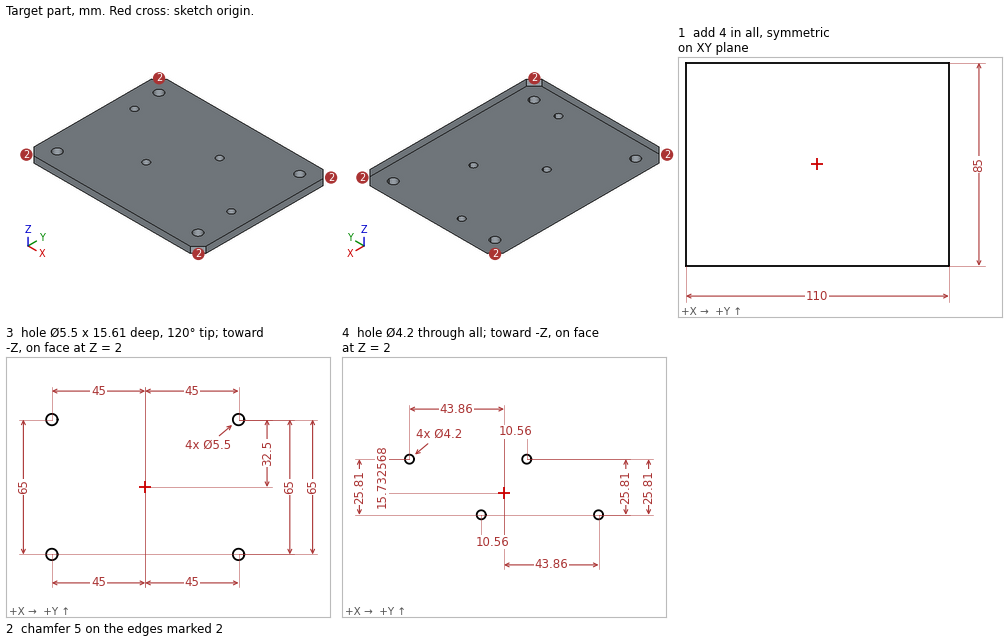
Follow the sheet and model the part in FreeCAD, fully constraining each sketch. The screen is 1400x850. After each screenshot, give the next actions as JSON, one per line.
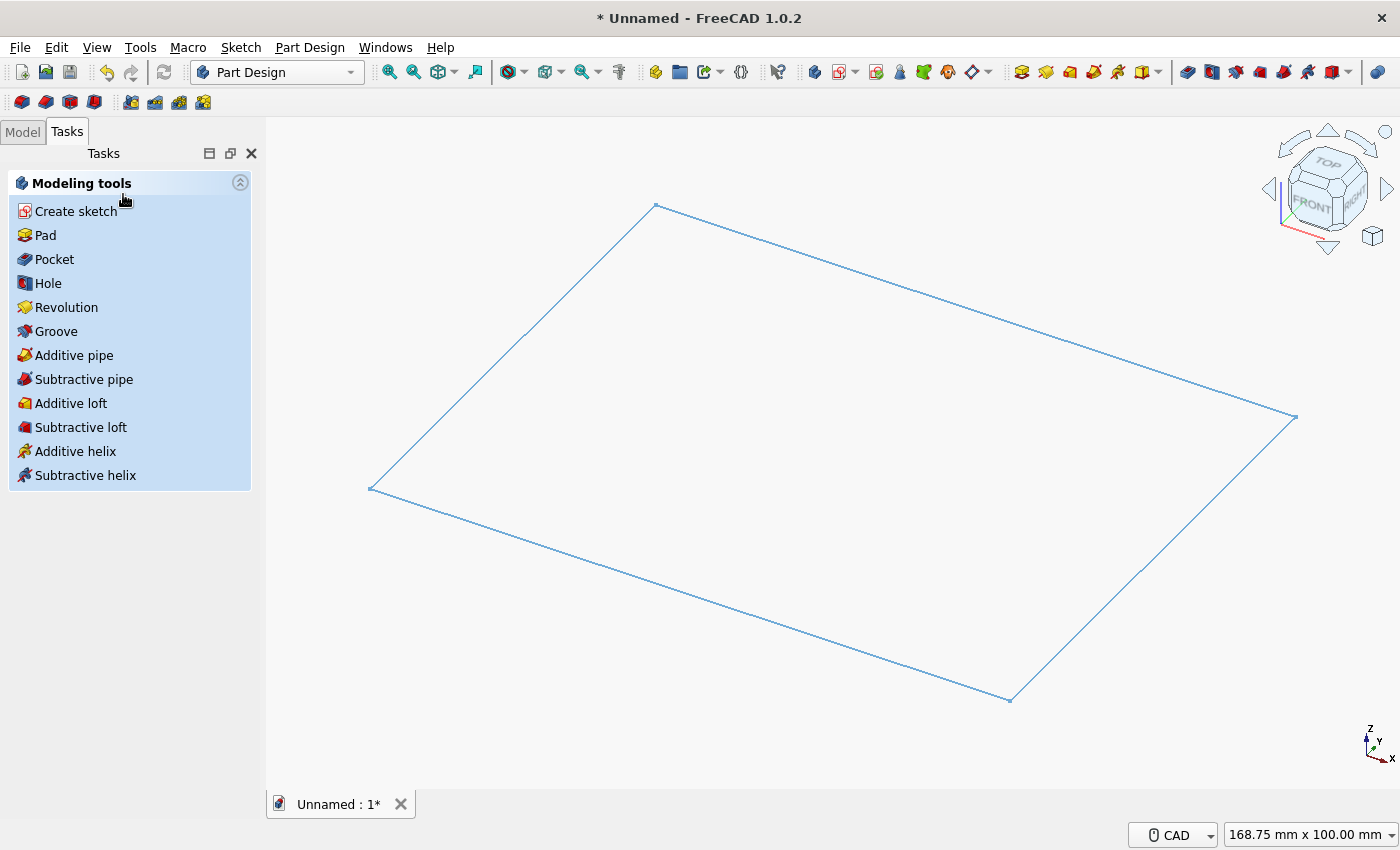
{"action": "left_click", "coordinate": [1022, 72]}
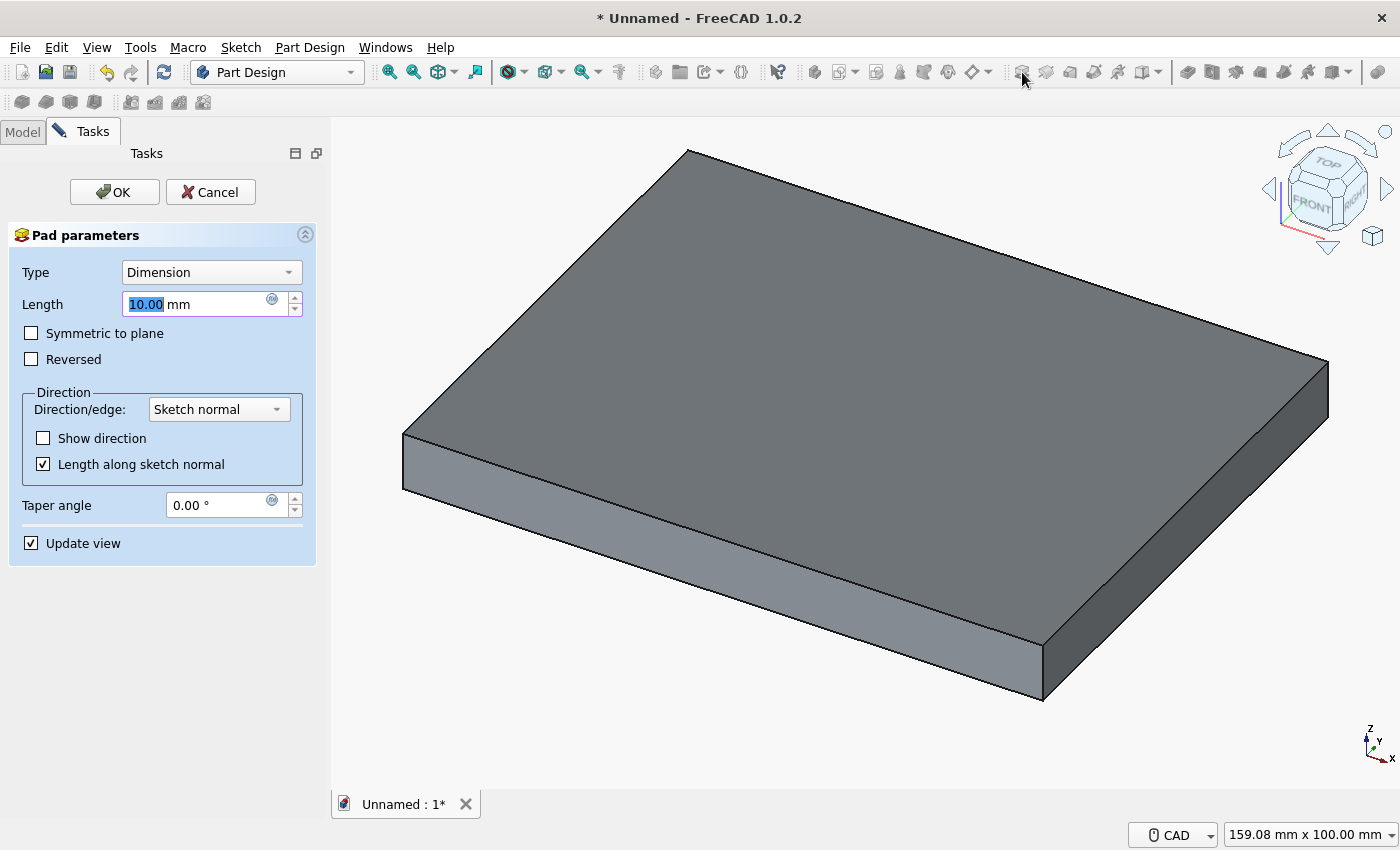
{"action": "type", "text": "4"}
{"action": "key", "text": "Tab"}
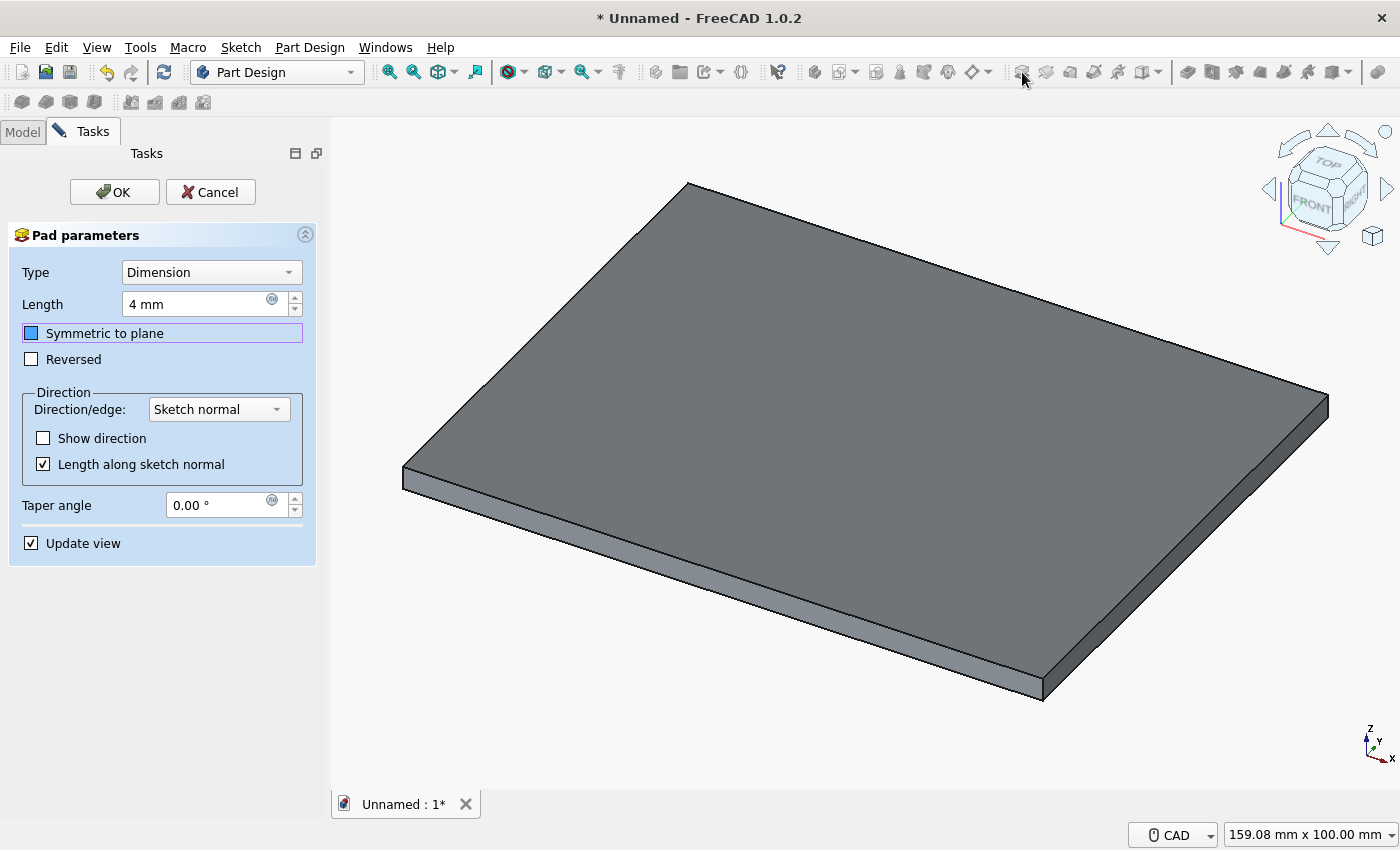
{"action": "left_click", "coordinate": [30, 333]}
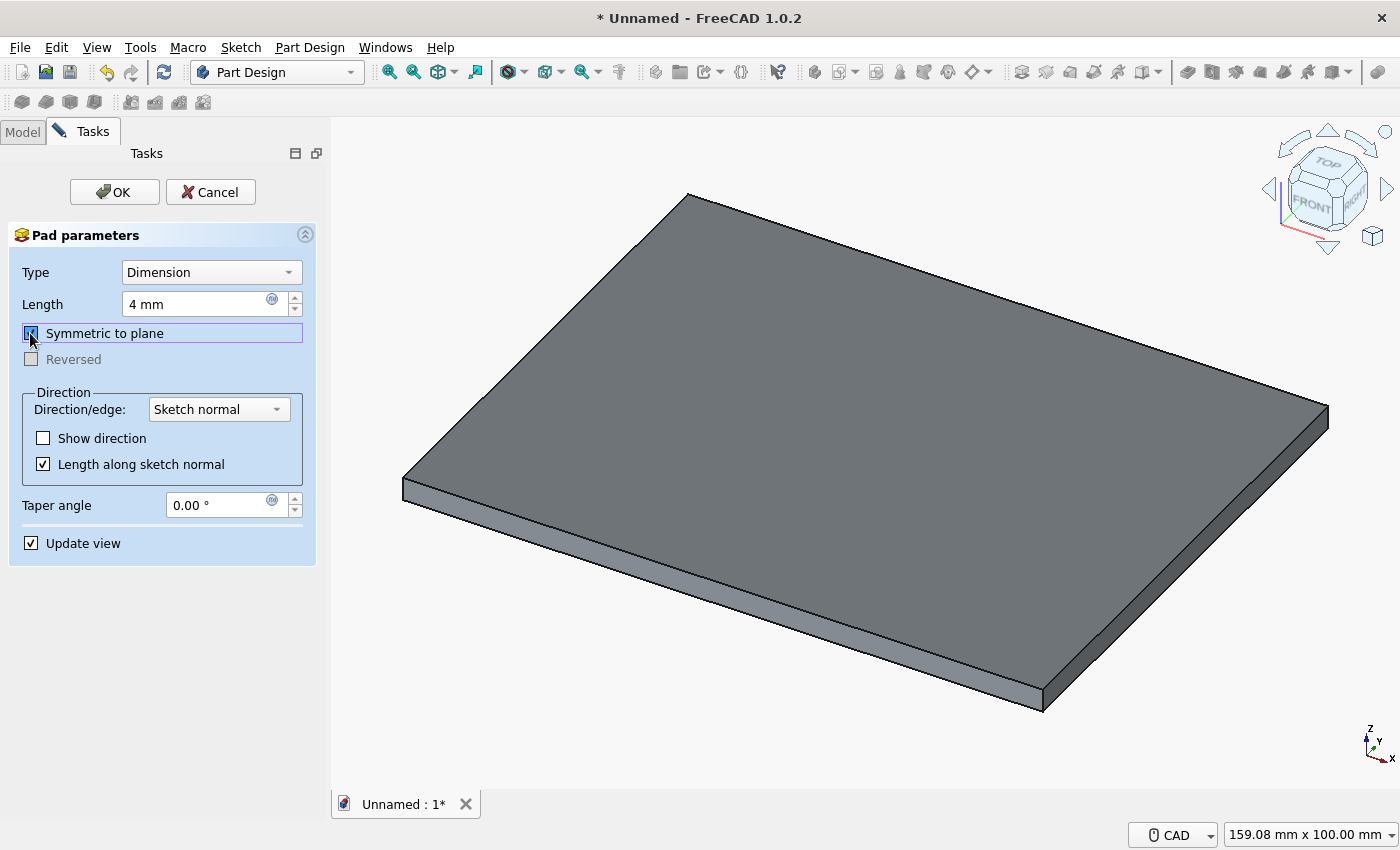
{"action": "left_click", "coordinate": [115, 192]}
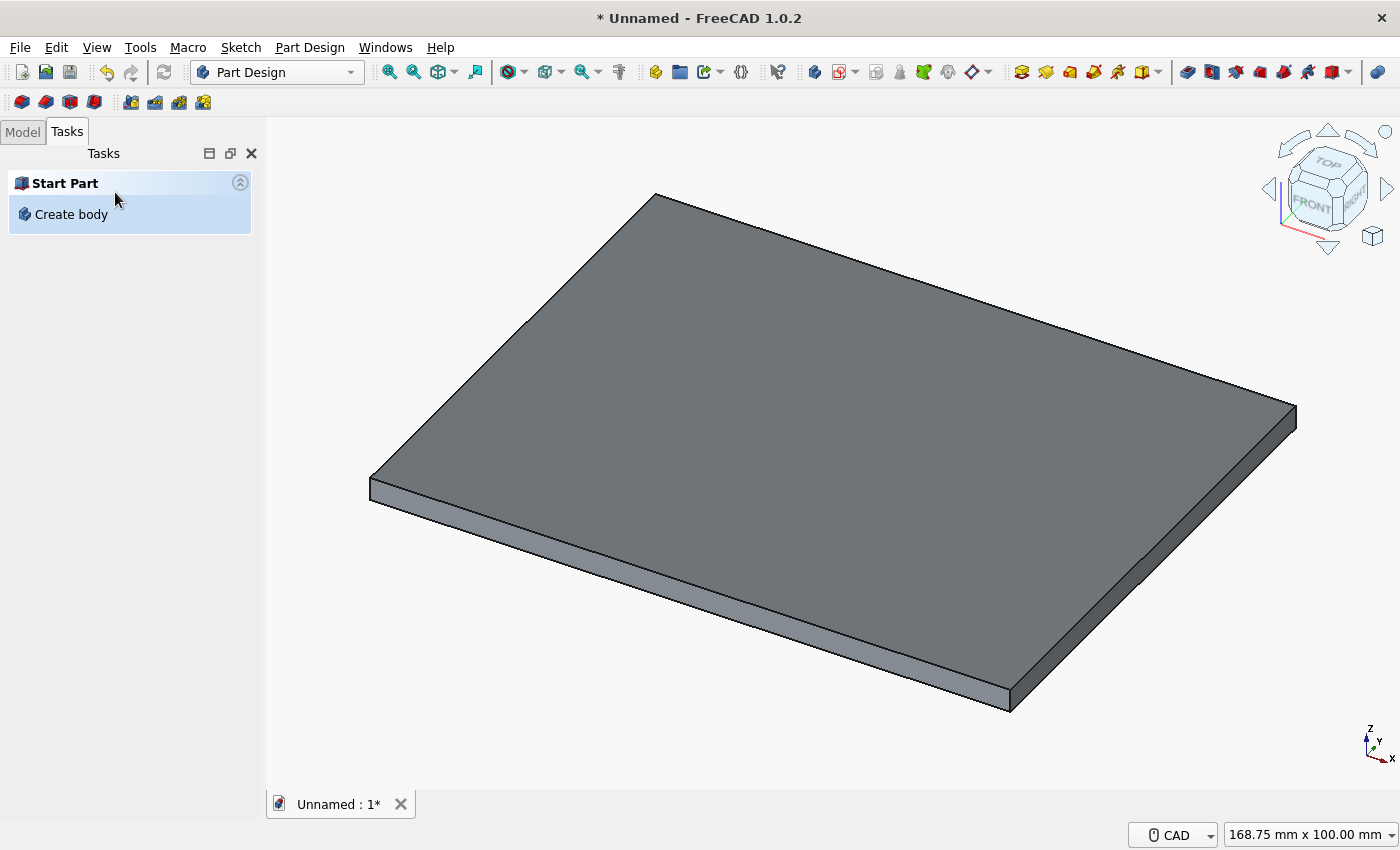
{"action": "left_click", "coordinate": [1010, 700]}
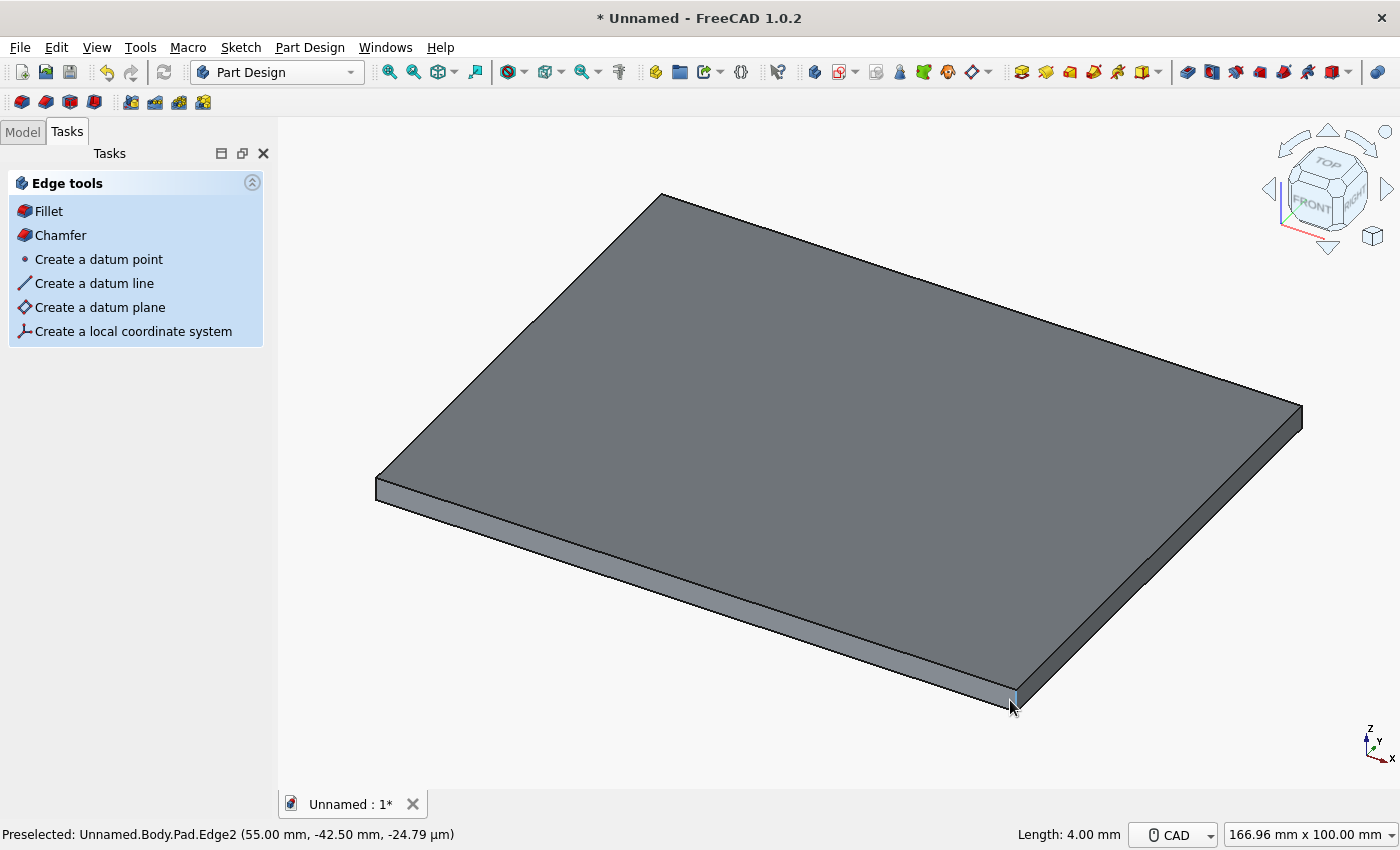
{"action": "key", "text": "0"}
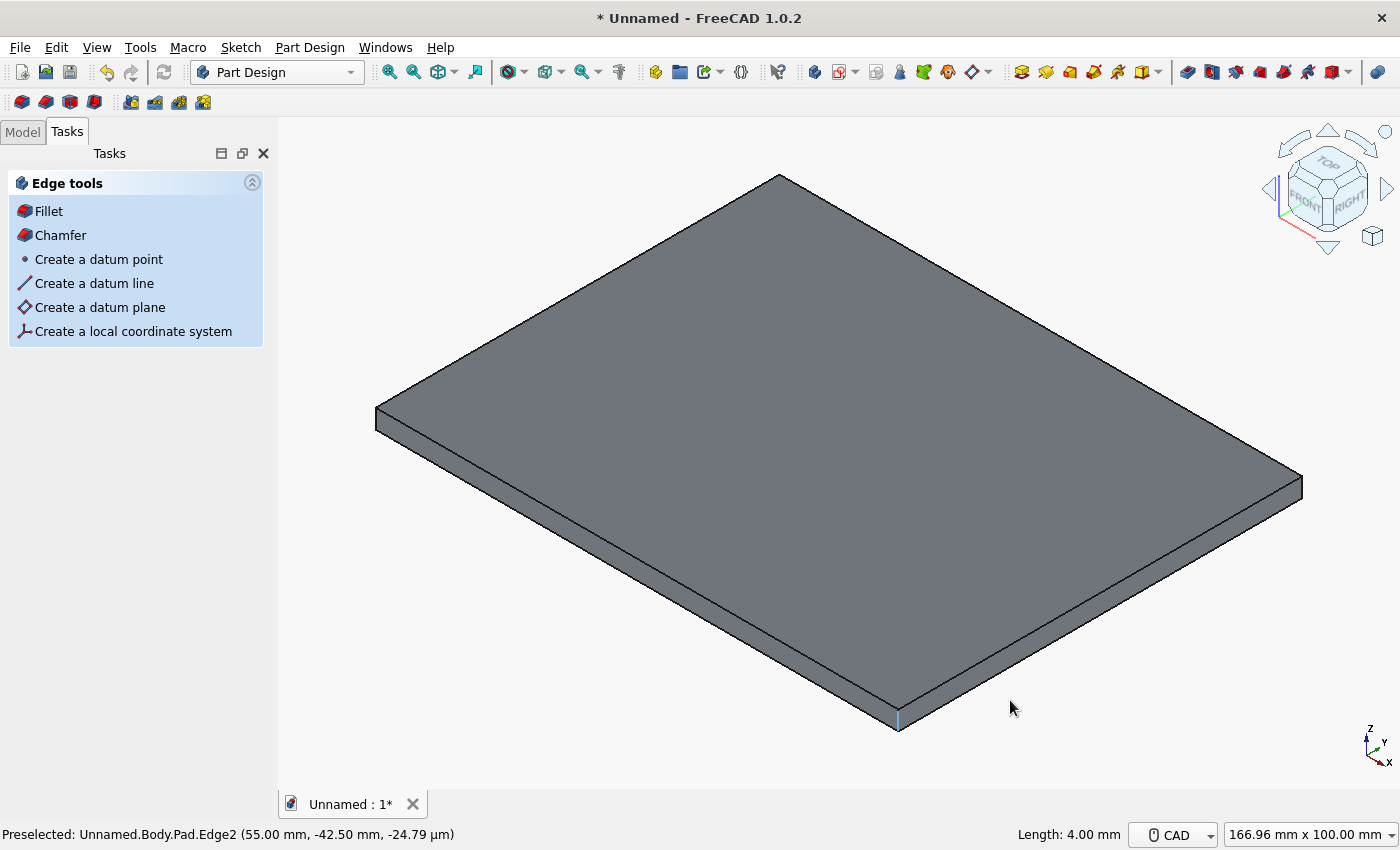
{"action": "key", "text": "2"}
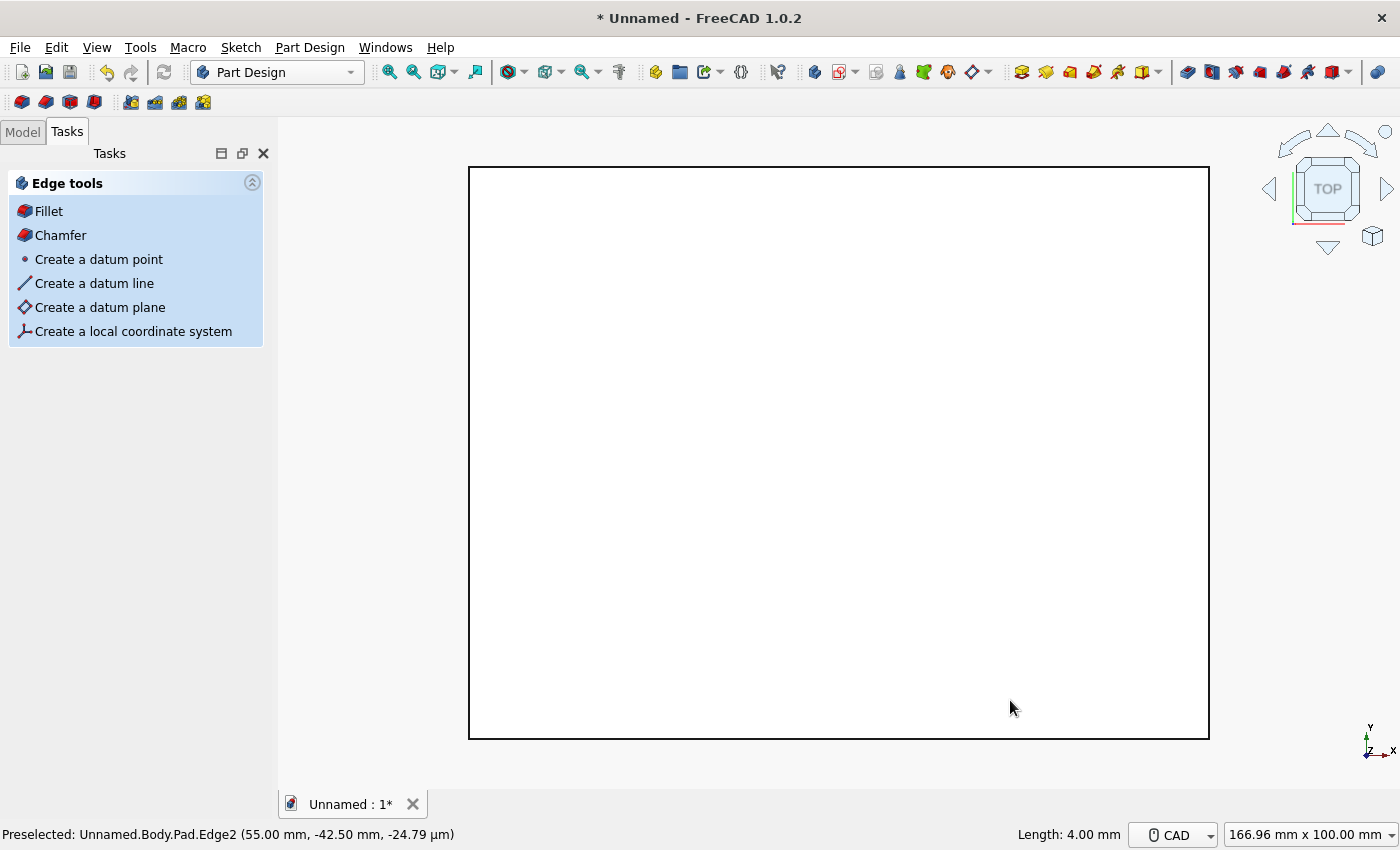
{"action": "key", "text": "1"}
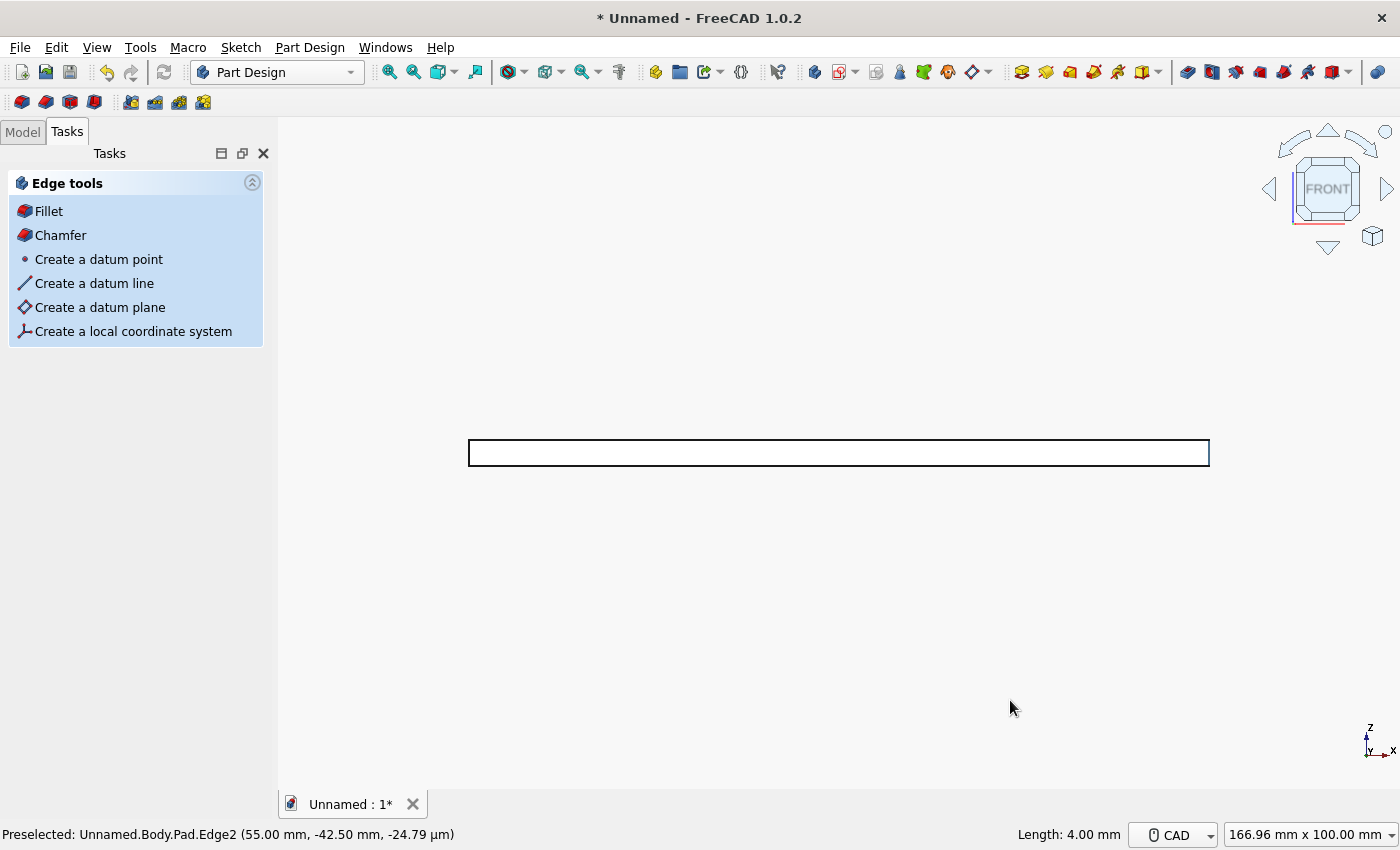
{"action": "left_click", "coordinate": [469, 452], "text": "ctrl"}